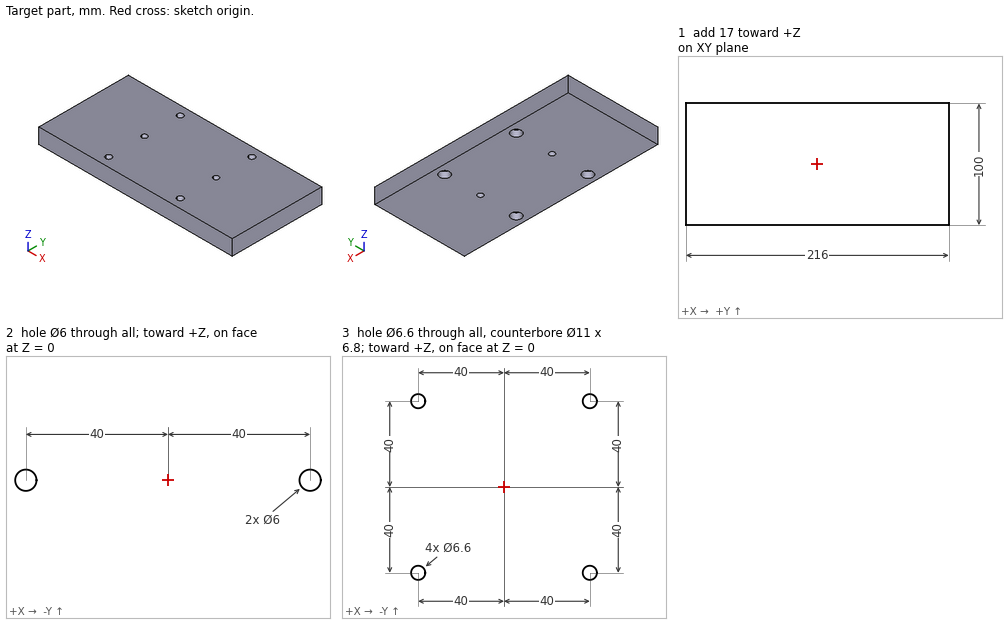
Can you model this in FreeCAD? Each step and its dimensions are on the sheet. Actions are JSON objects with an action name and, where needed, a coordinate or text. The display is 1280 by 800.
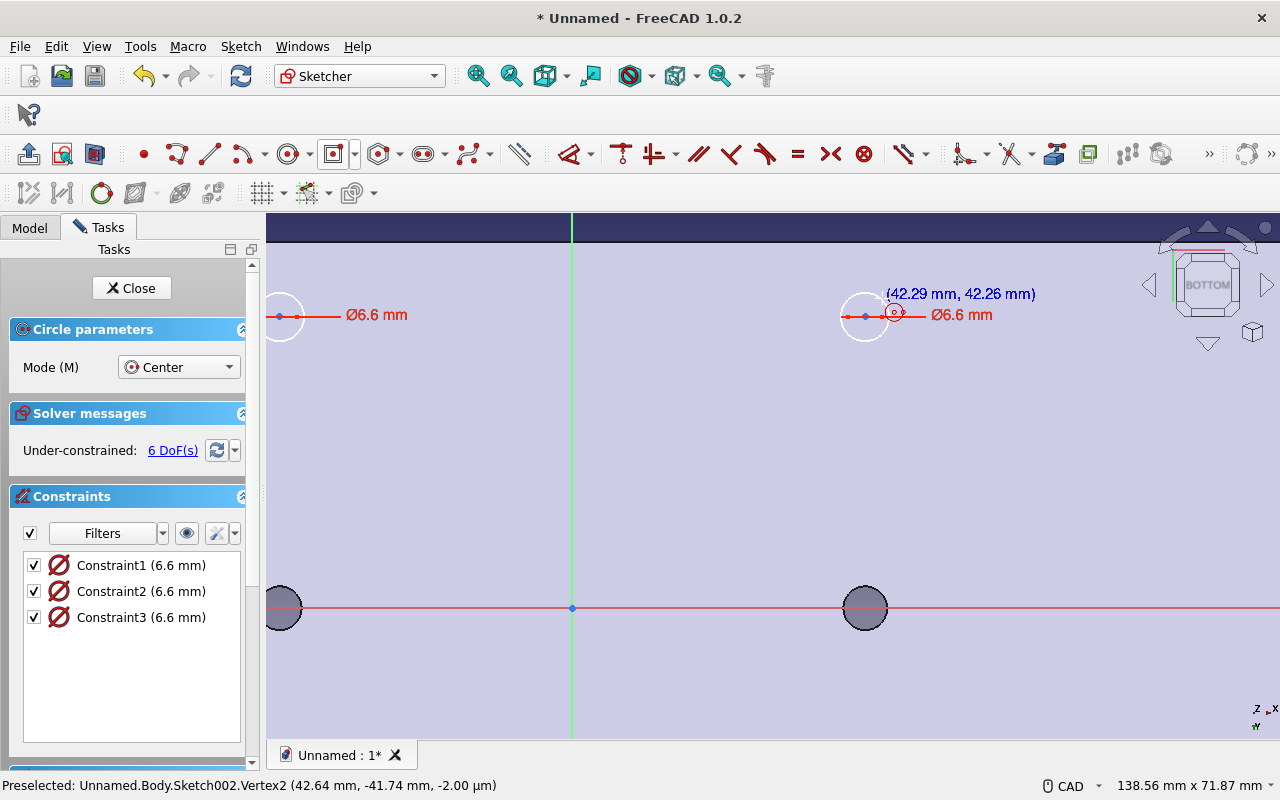
{"action": "scroll", "coordinate": [865, 315], "scroll_direction": "down", "scroll_amount": 3}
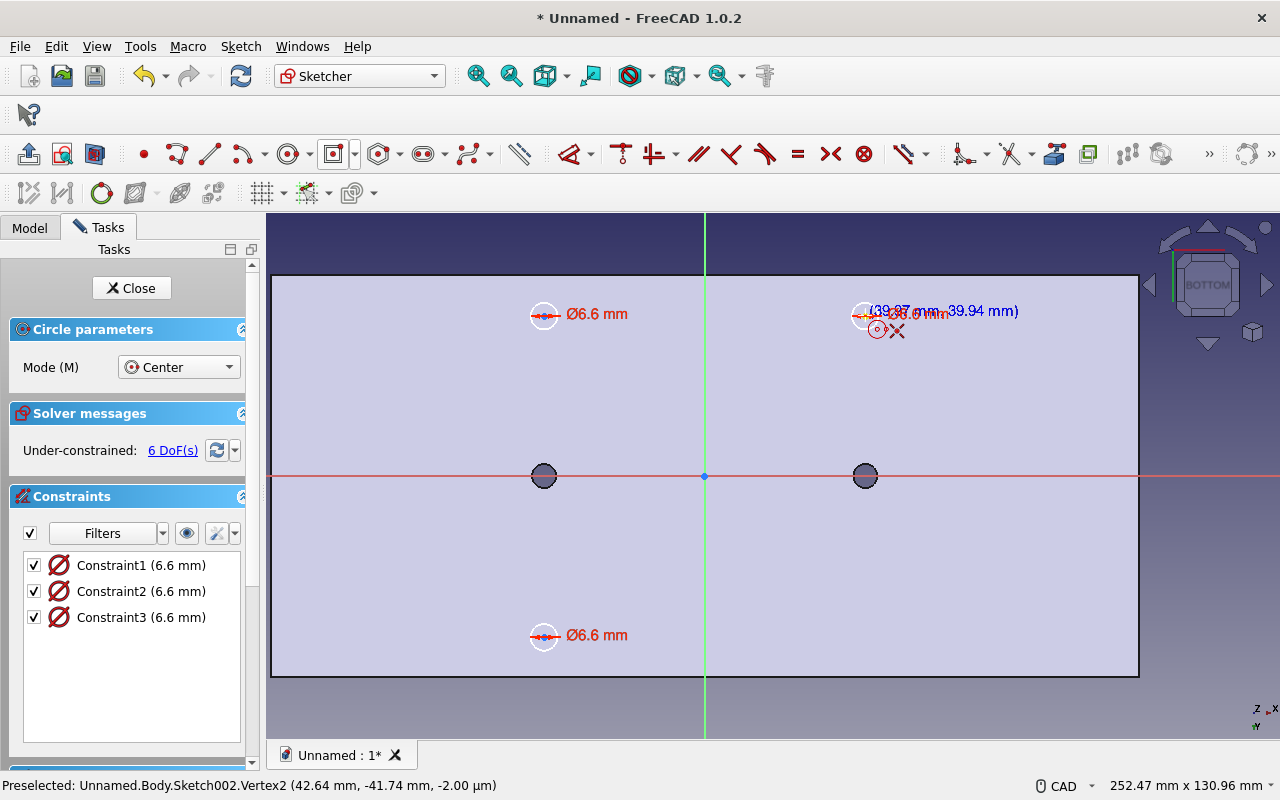
{"action": "scroll", "coordinate": [865, 637], "scroll_direction": "up", "scroll_amount": 3}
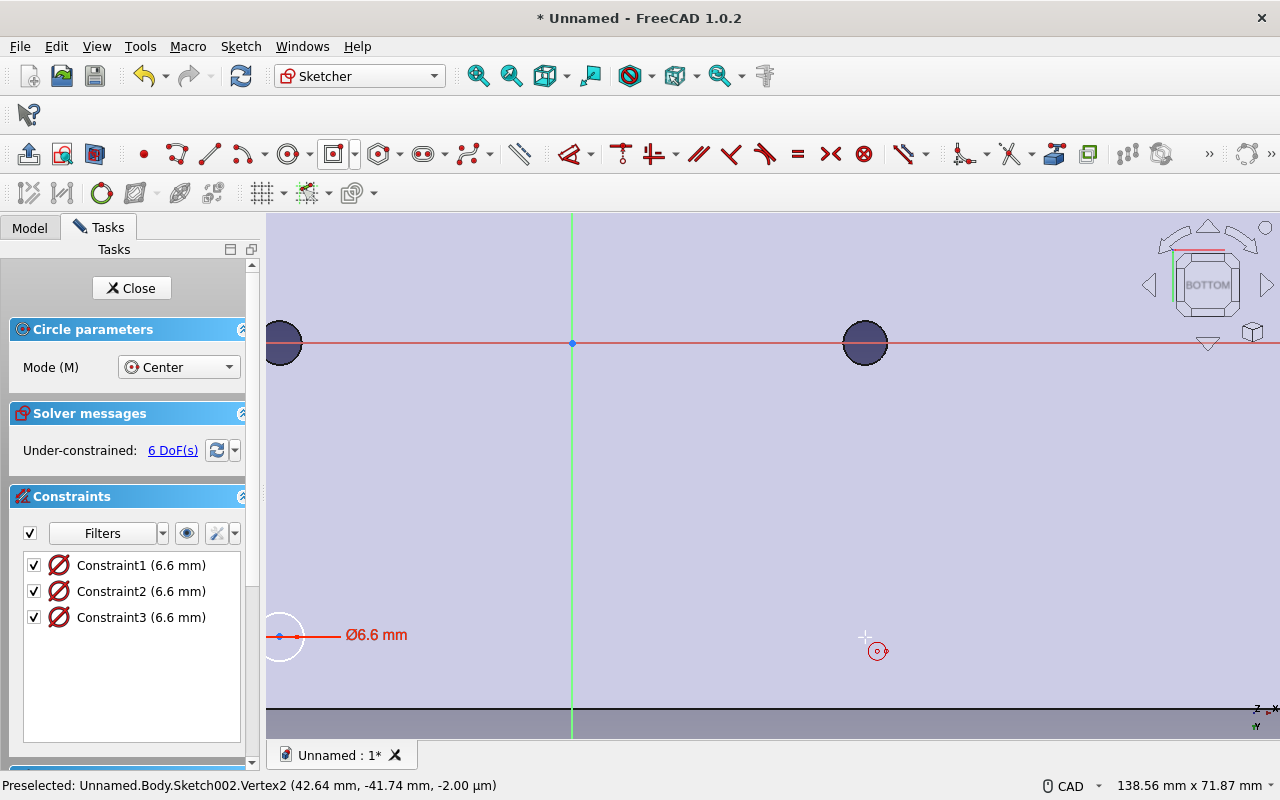
{"action": "left_click", "coordinate": [865, 636]}
{"action": "mouse_move", "coordinate": [882, 619]}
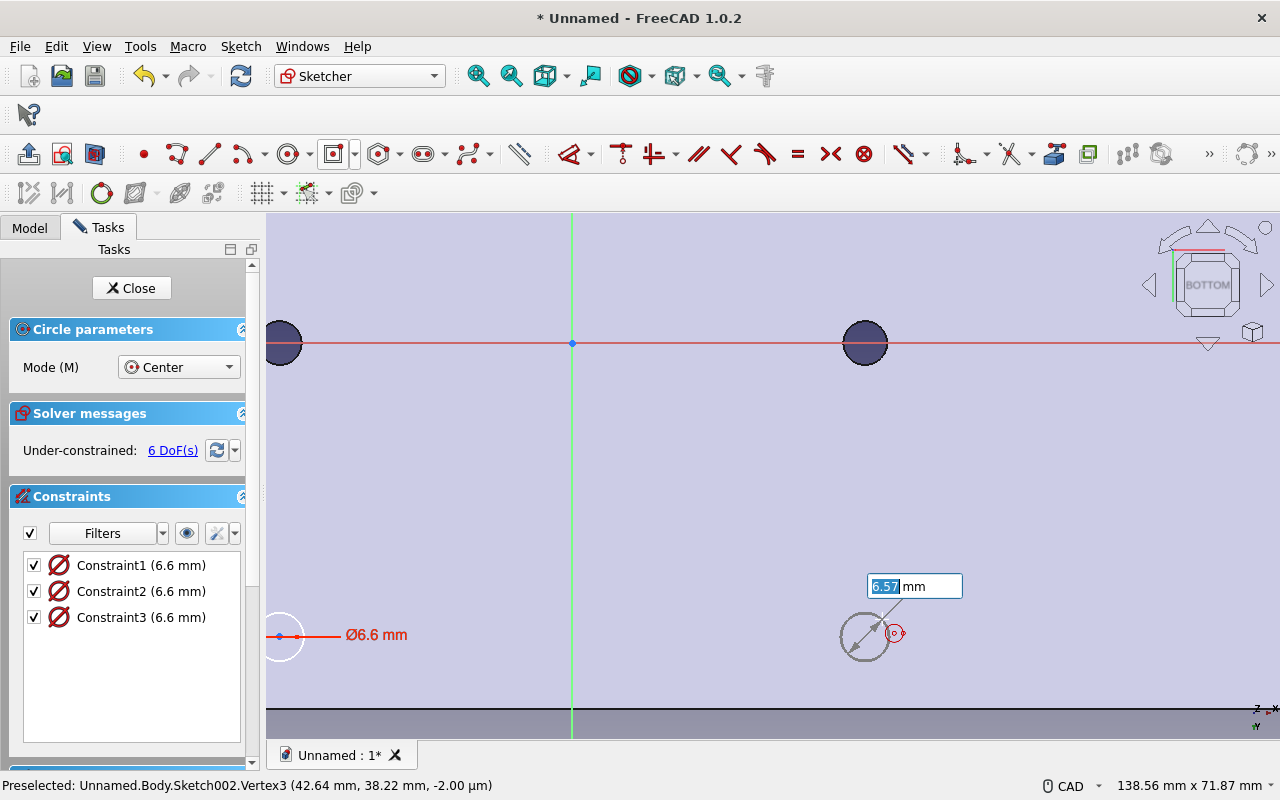
{"action": "type", "text": "6.6"}
{"action": "key", "text": "Return"}
{"action": "key", "text": "Escape"}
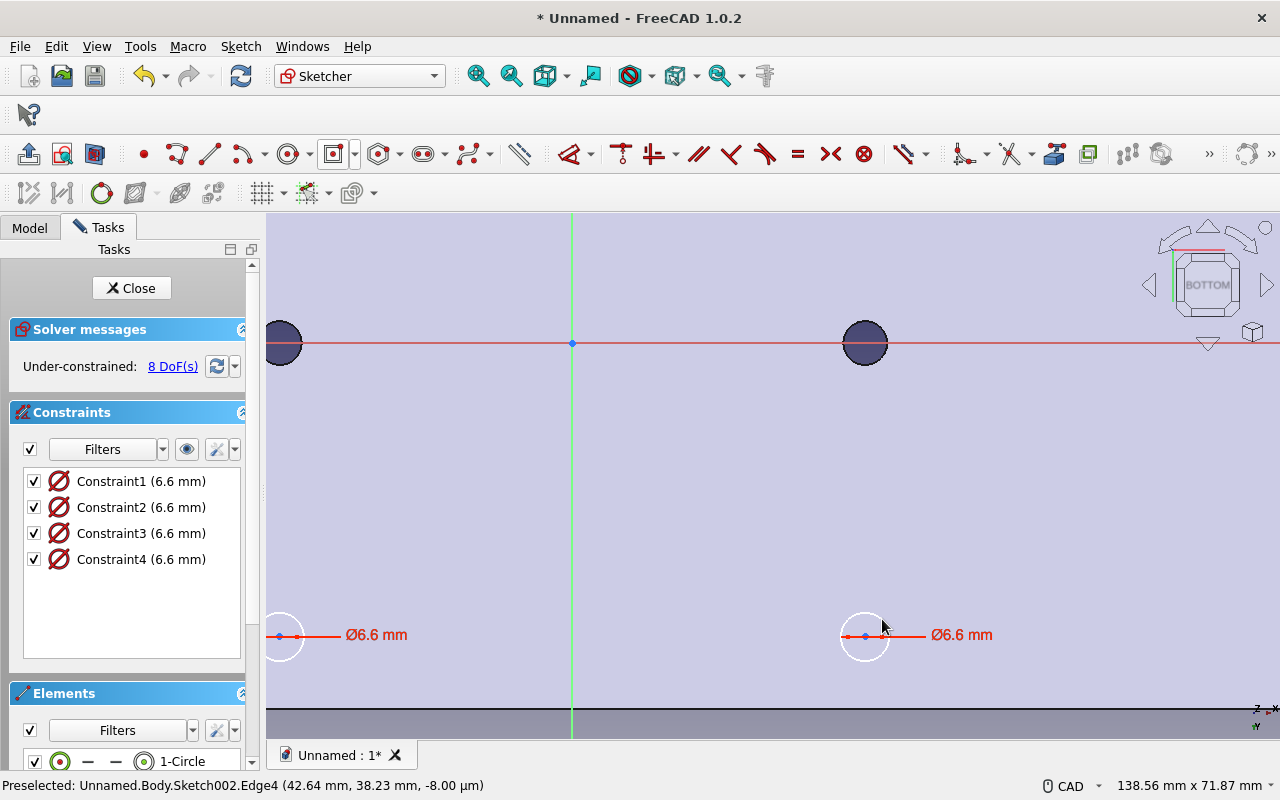
{"action": "left_click", "coordinate": [568, 154]}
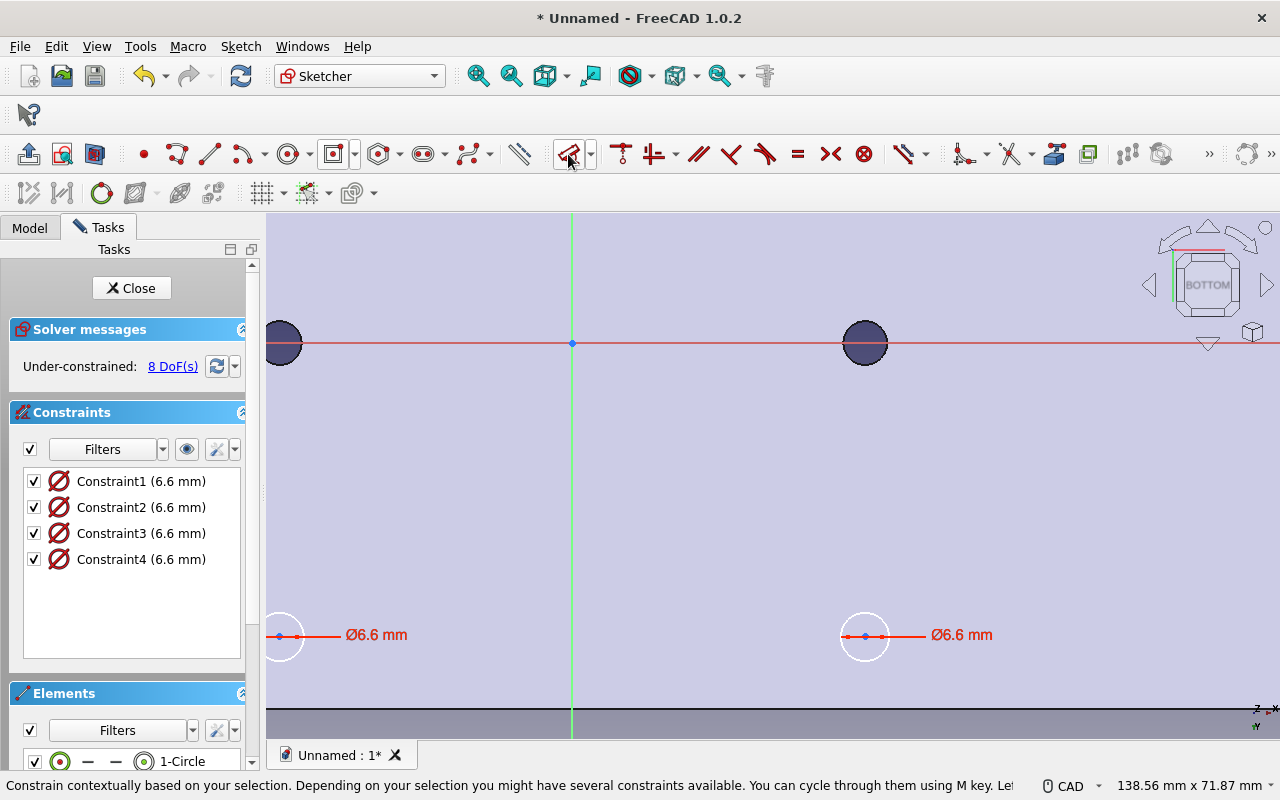
{"action": "scroll", "coordinate": [865, 638], "scroll_direction": "down", "scroll_amount": 3}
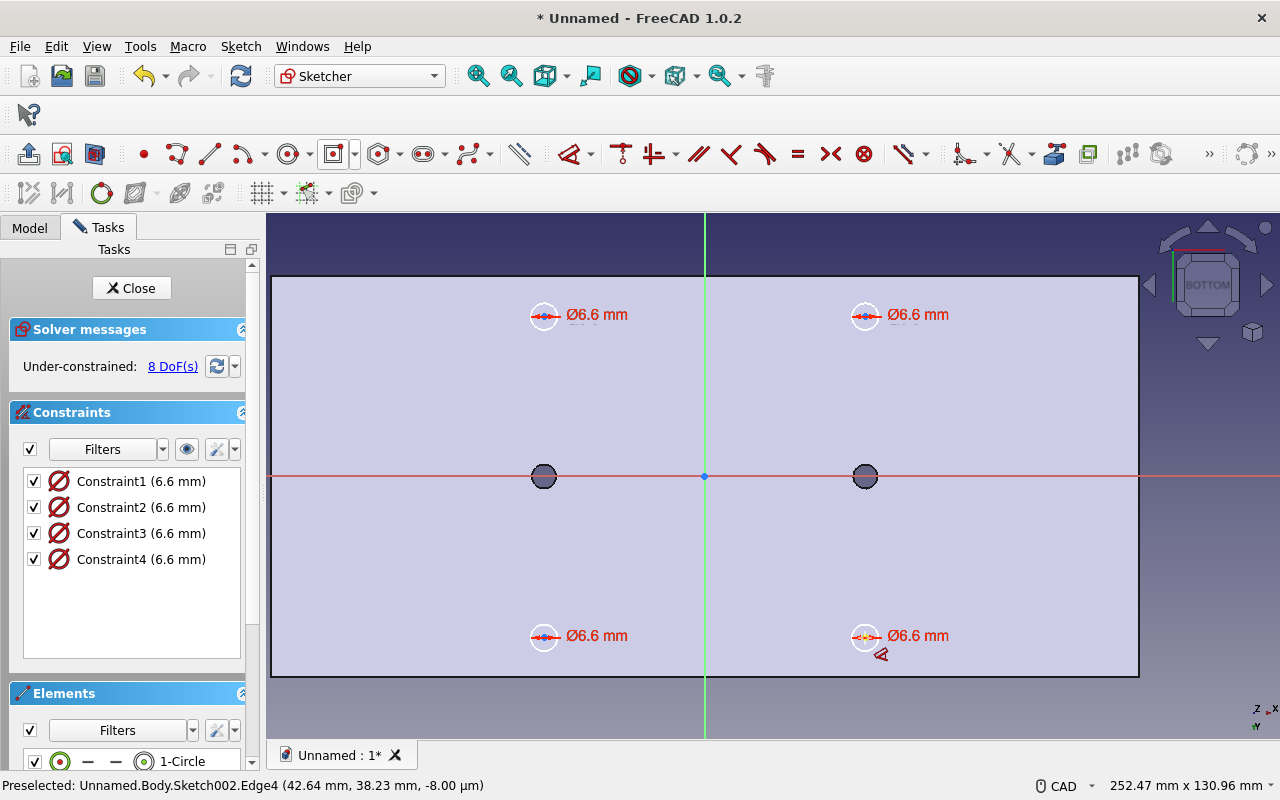
{"action": "left_click", "coordinate": [544, 638]}
{"action": "left_click", "coordinate": [624, 672]}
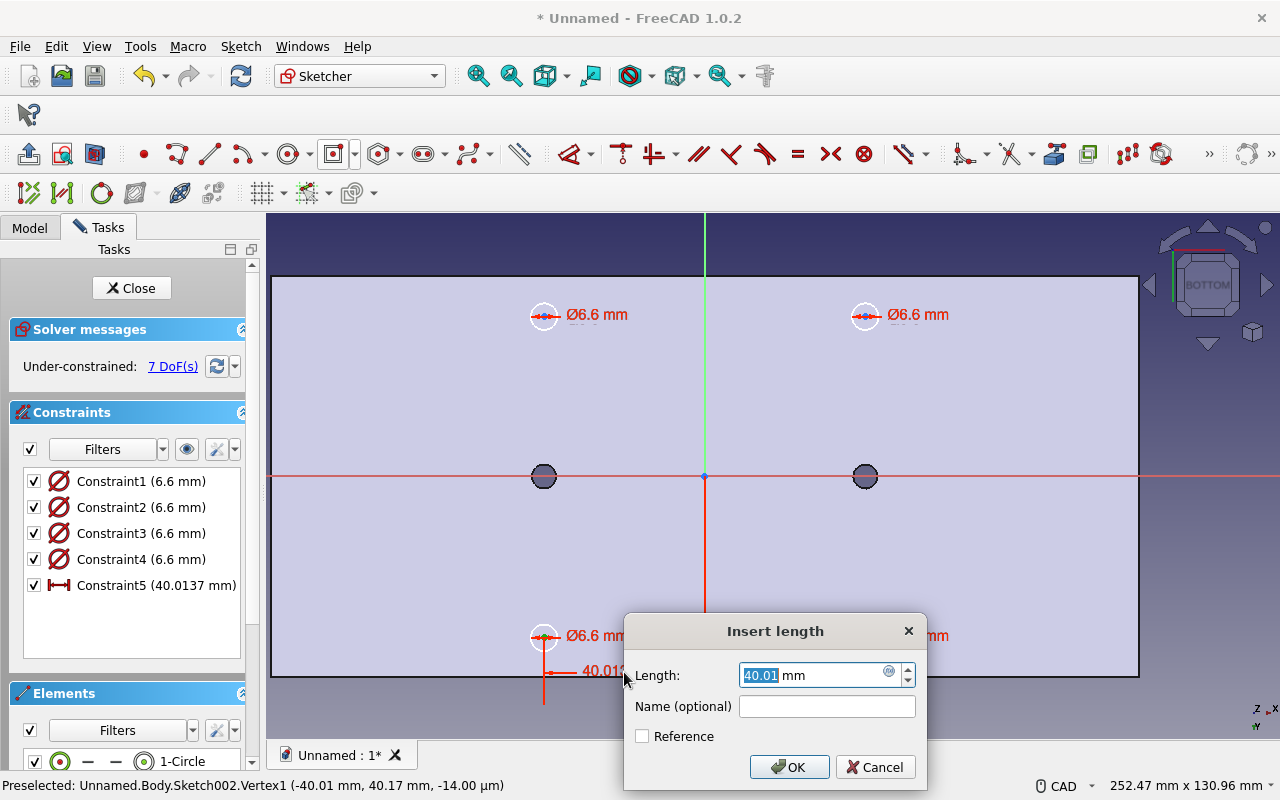
{"action": "type", "text": "40"}
{"action": "key", "text": "Return"}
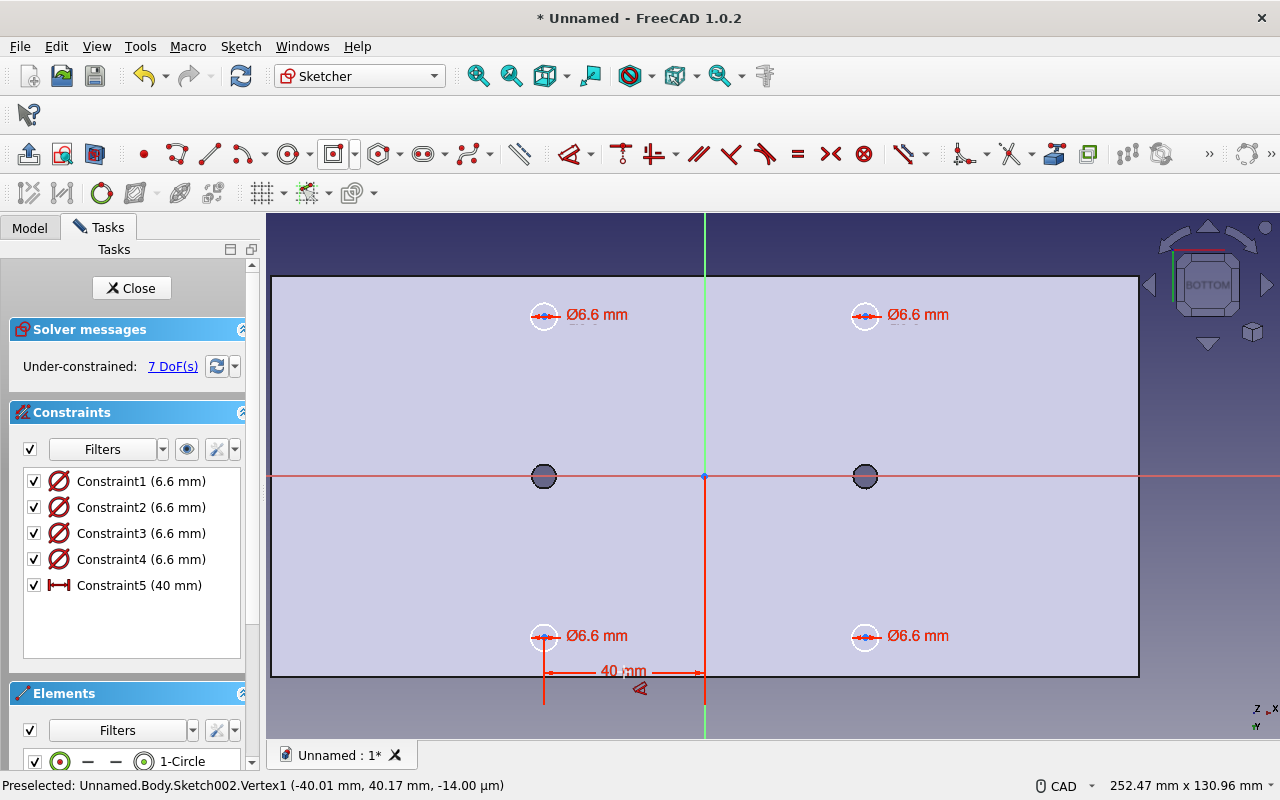
{"action": "left_click", "coordinate": [544, 638]}
{"action": "left_click", "coordinate": [510, 557]}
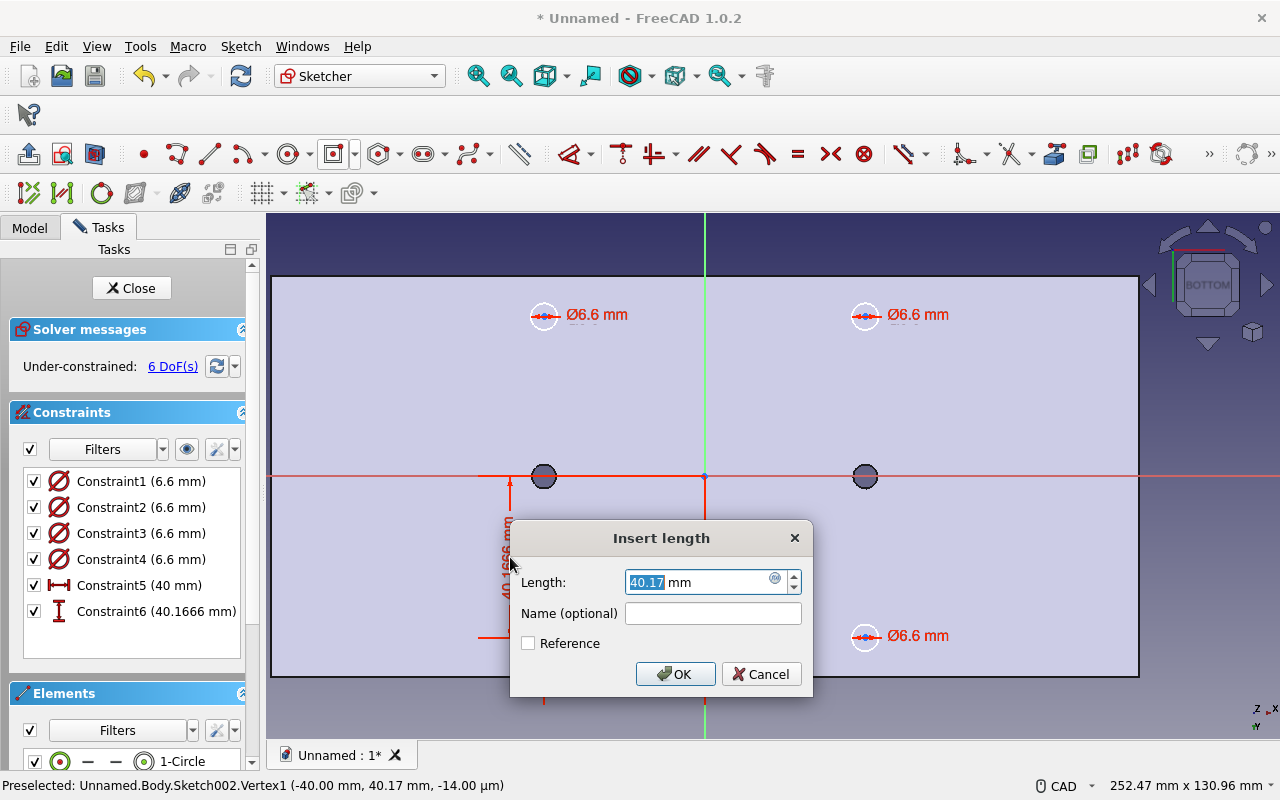
{"action": "type", "text": "40"}
{"action": "key", "text": "Return"}